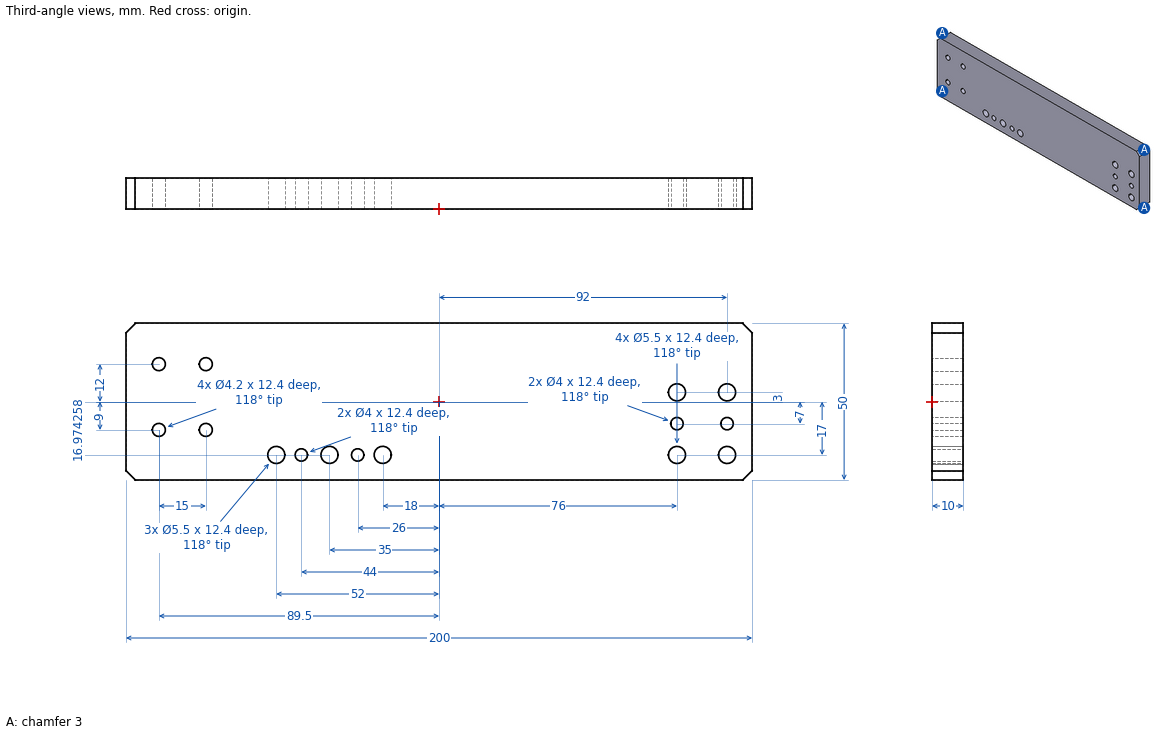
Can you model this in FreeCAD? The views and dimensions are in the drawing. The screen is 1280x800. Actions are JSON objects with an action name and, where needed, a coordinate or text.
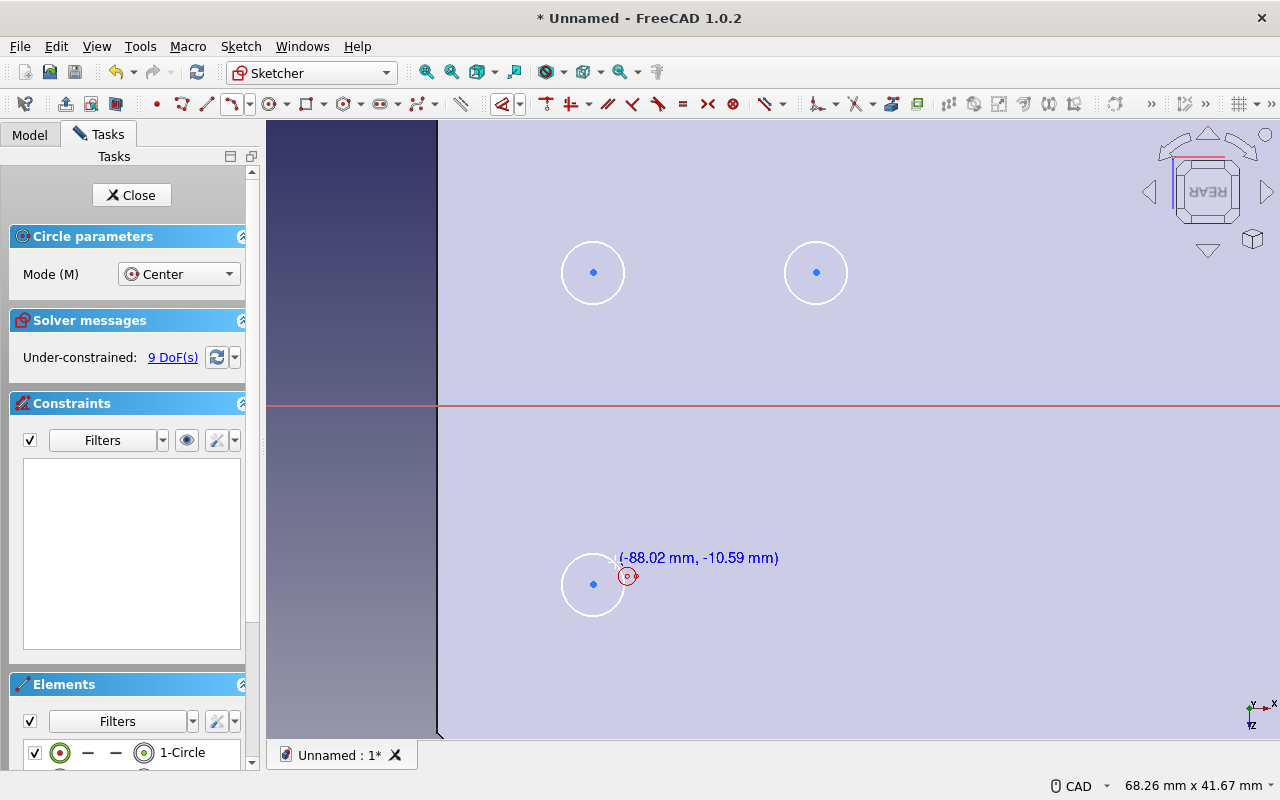
{"action": "left_click", "coordinate": [816, 584]}
{"action": "left_click", "coordinate": [838, 562]}
{"action": "key", "text": "Escape"}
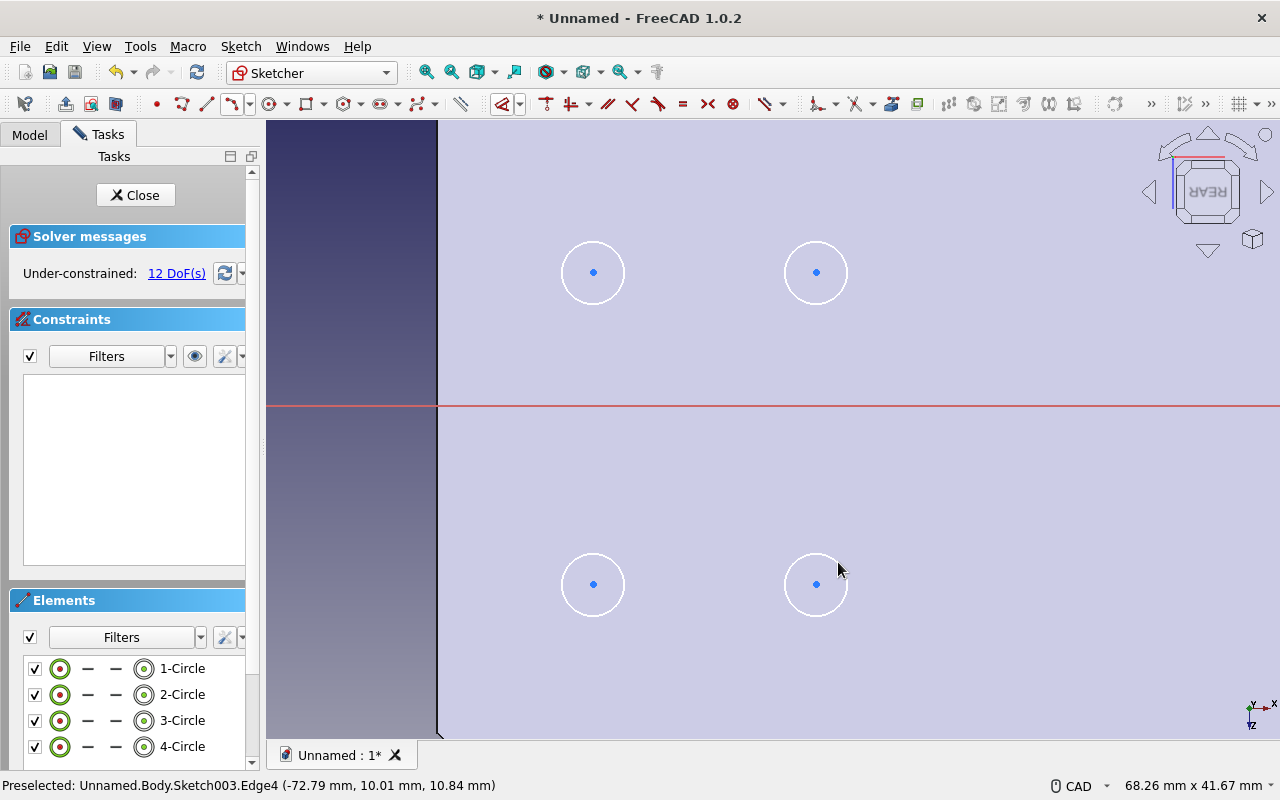
{"action": "left_click", "coordinate": [615, 251]}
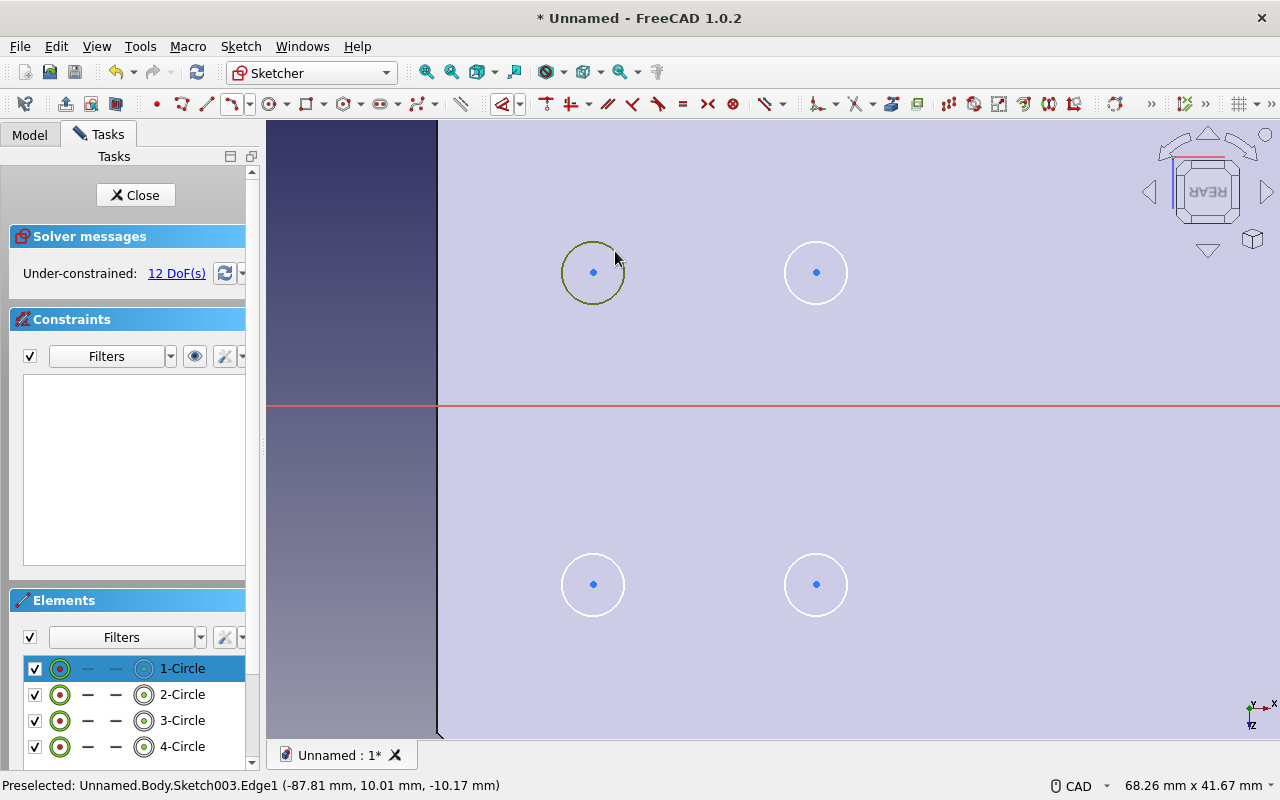
{"action": "left_click", "coordinate": [838, 251]}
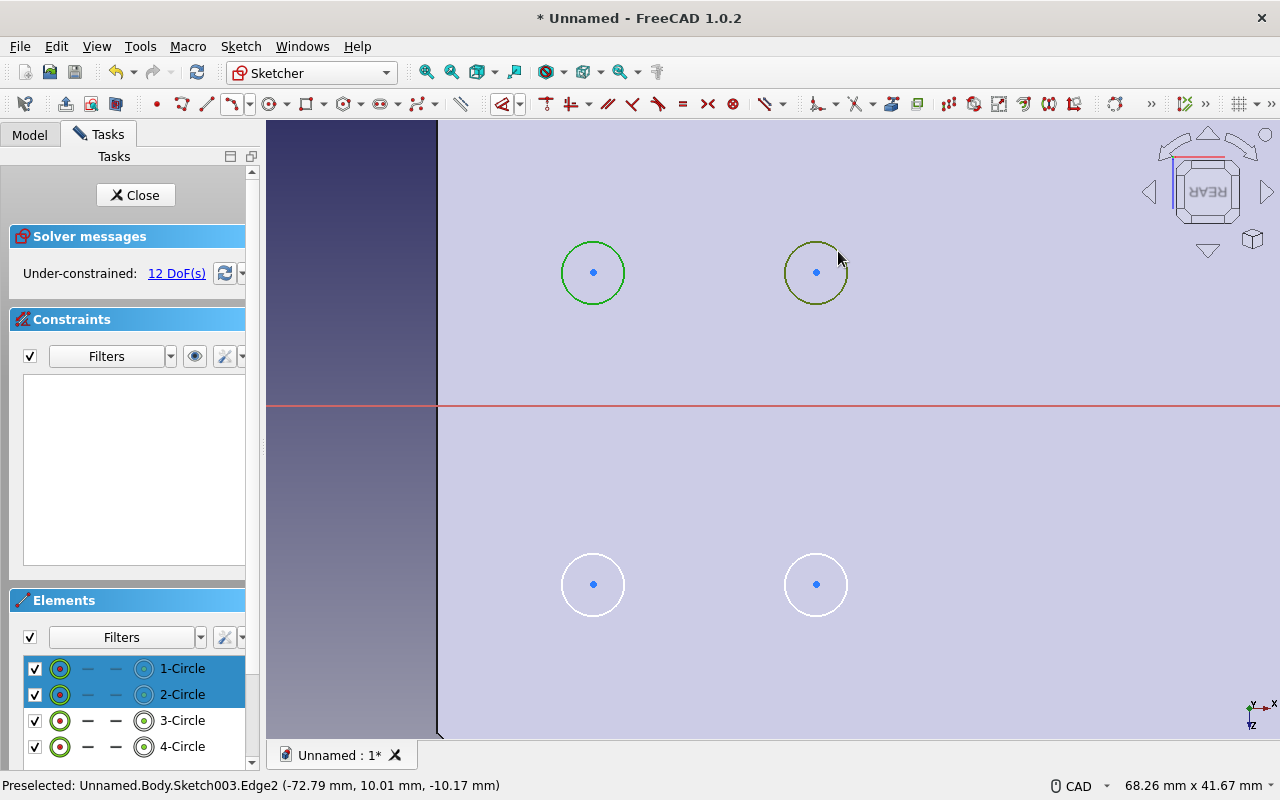
{"action": "left_click", "coordinate": [615, 563]}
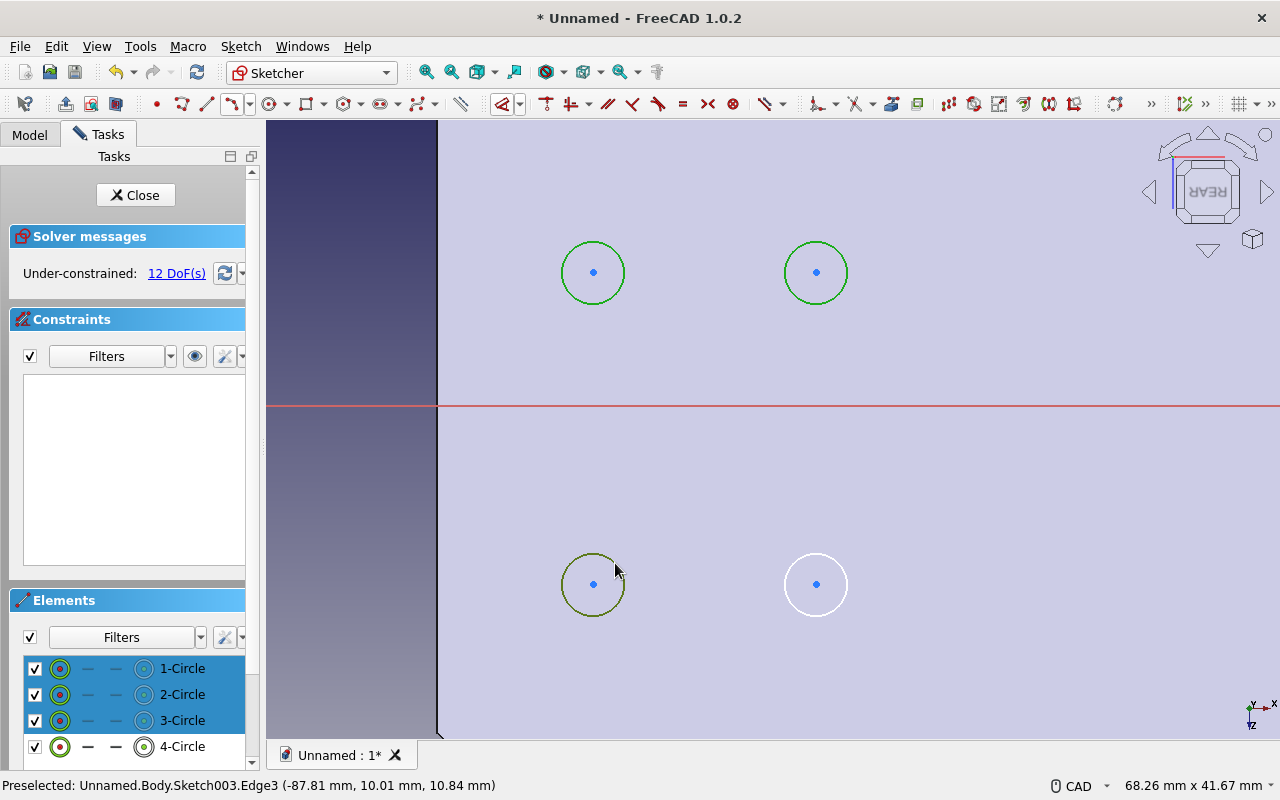
{"action": "left_click", "coordinate": [838, 563]}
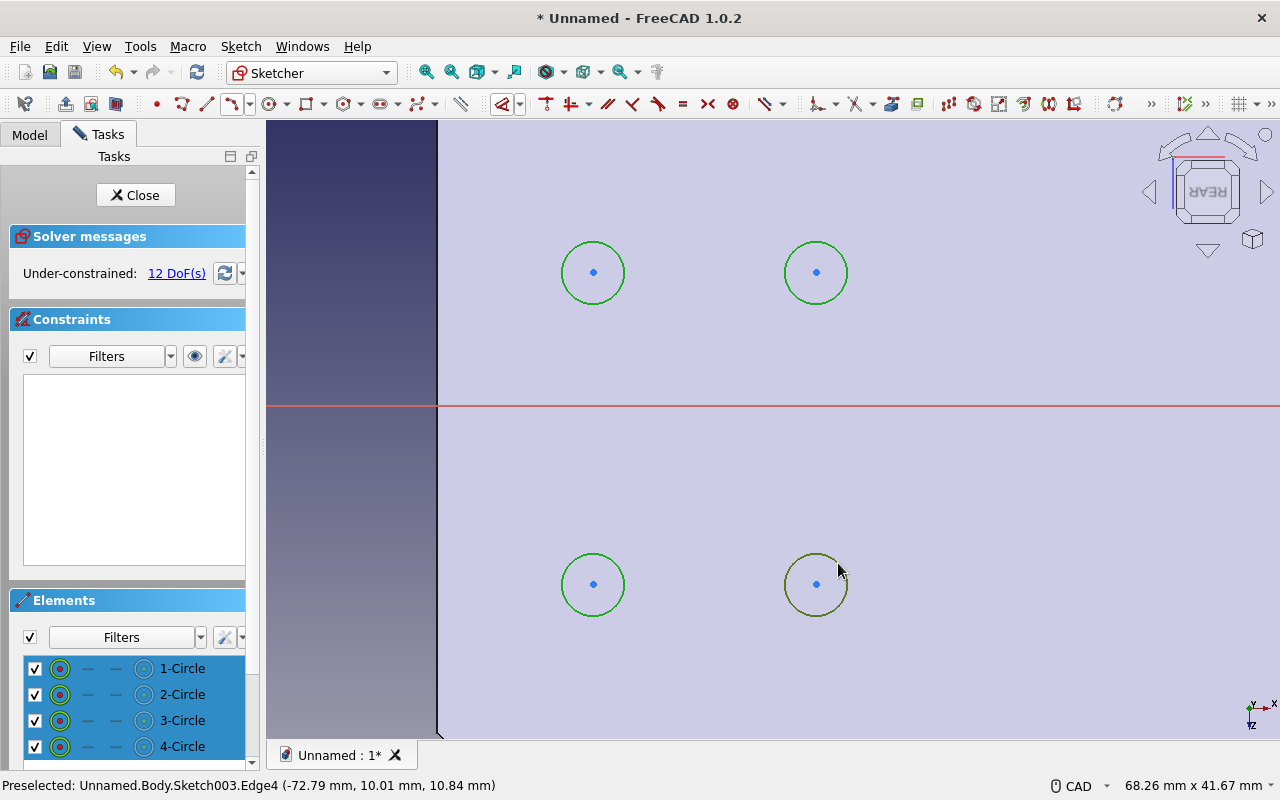
{"action": "left_click", "coordinate": [683, 104]}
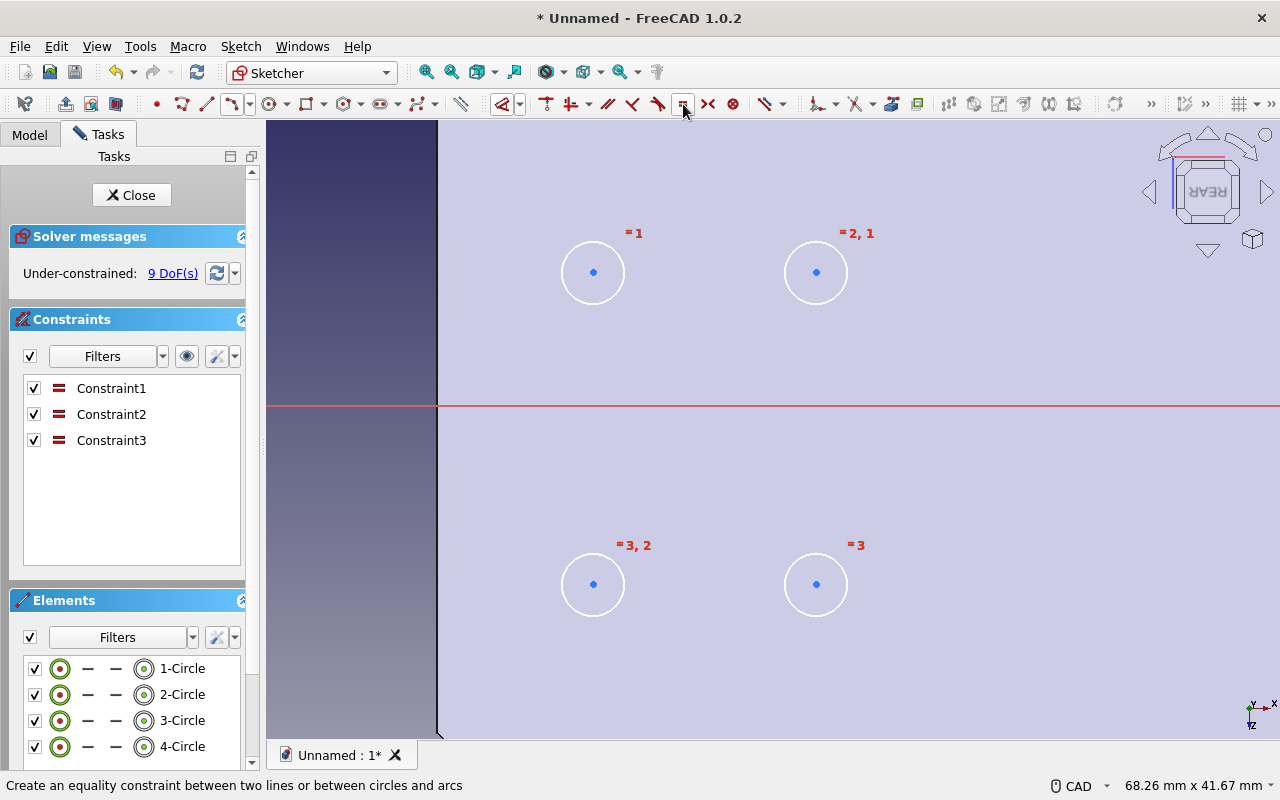
{"action": "left_click", "coordinate": [593, 273]}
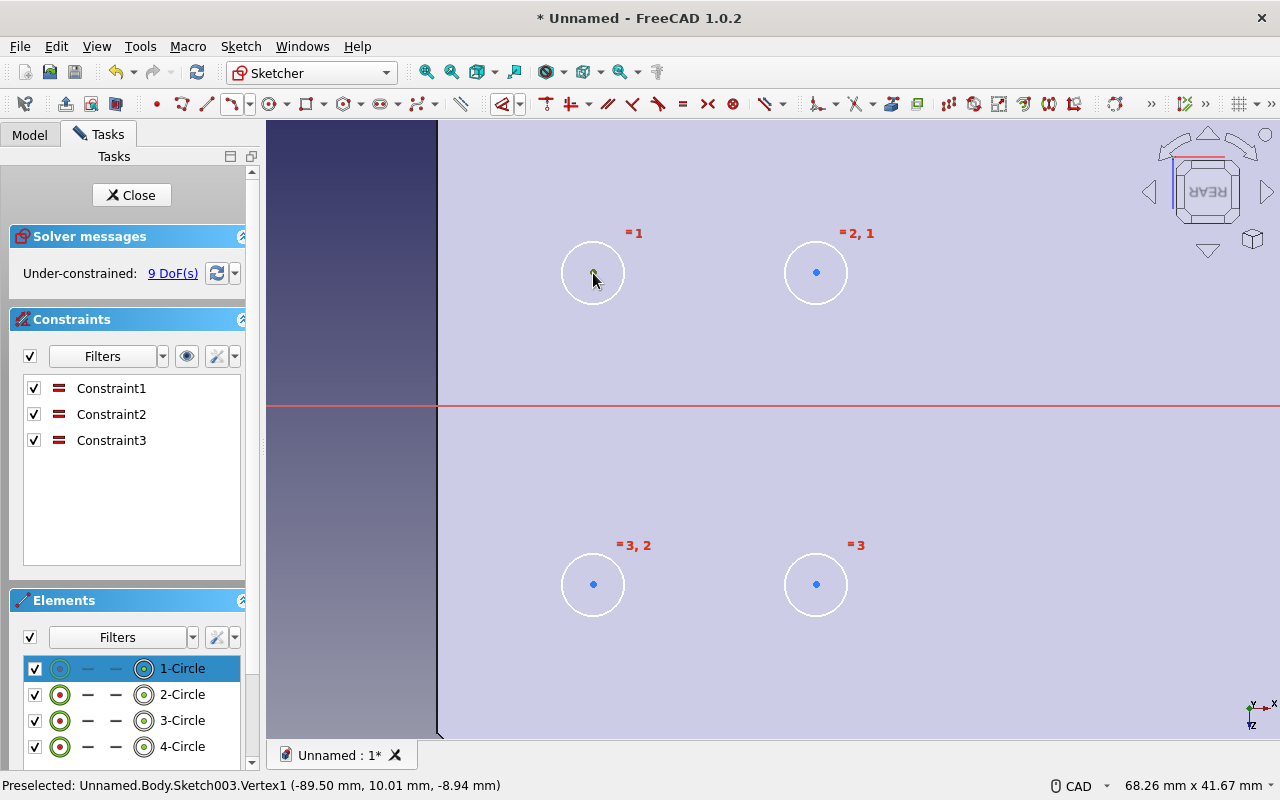
{"action": "left_click", "coordinate": [816, 273]}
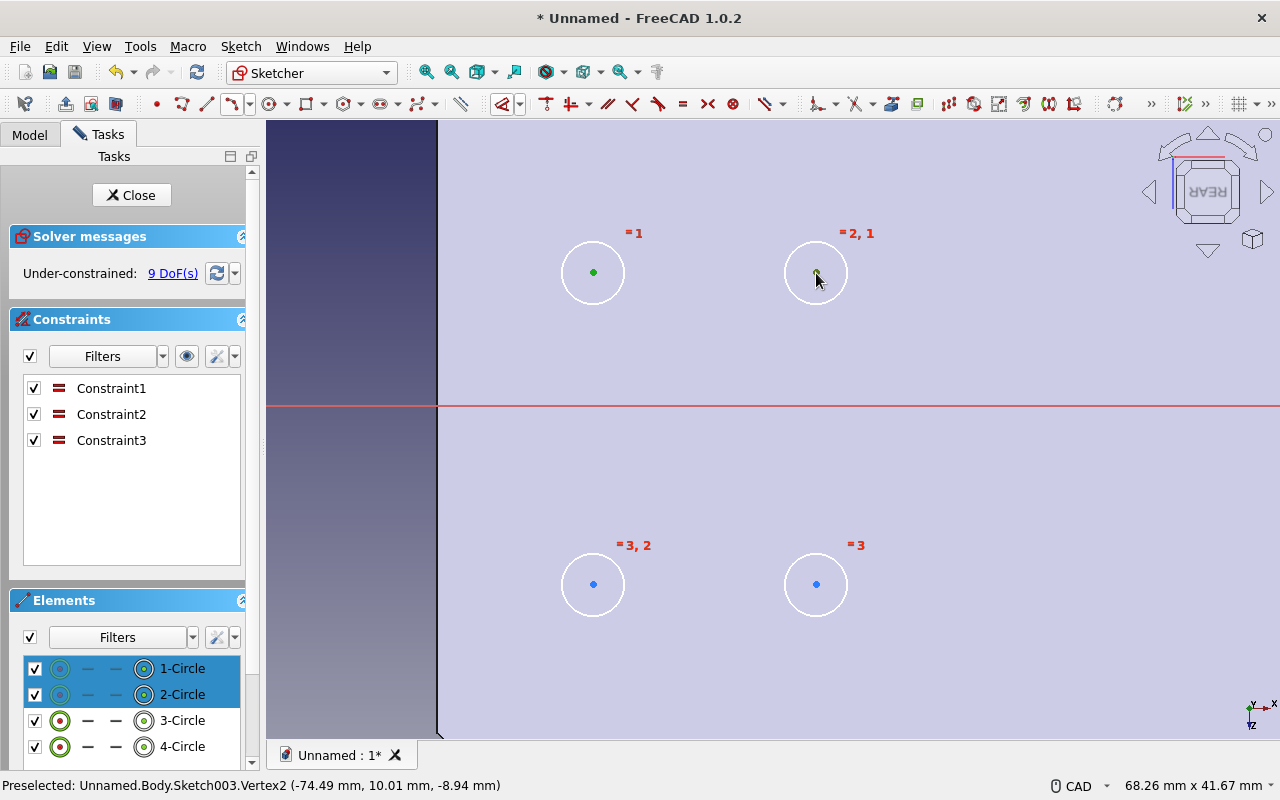
{"action": "key", "text": "h"}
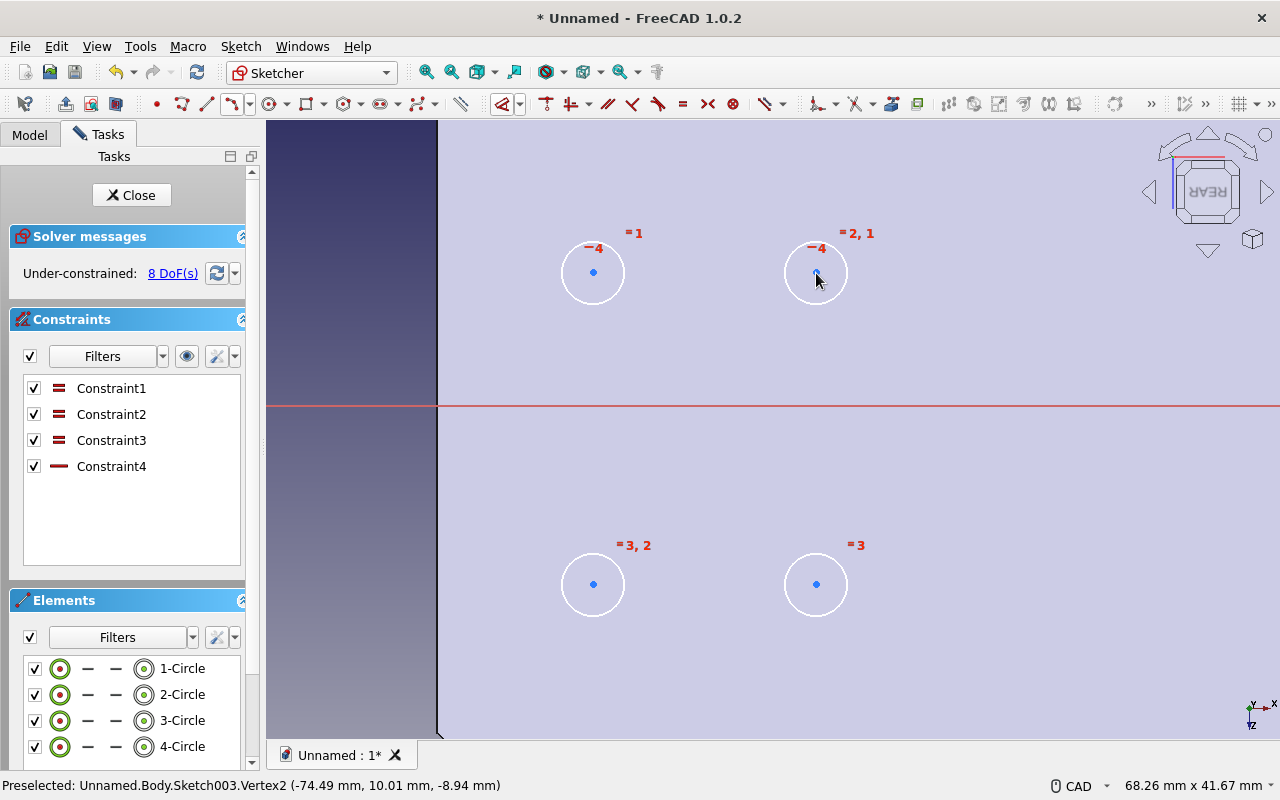
{"action": "left_click", "coordinate": [593, 273]}